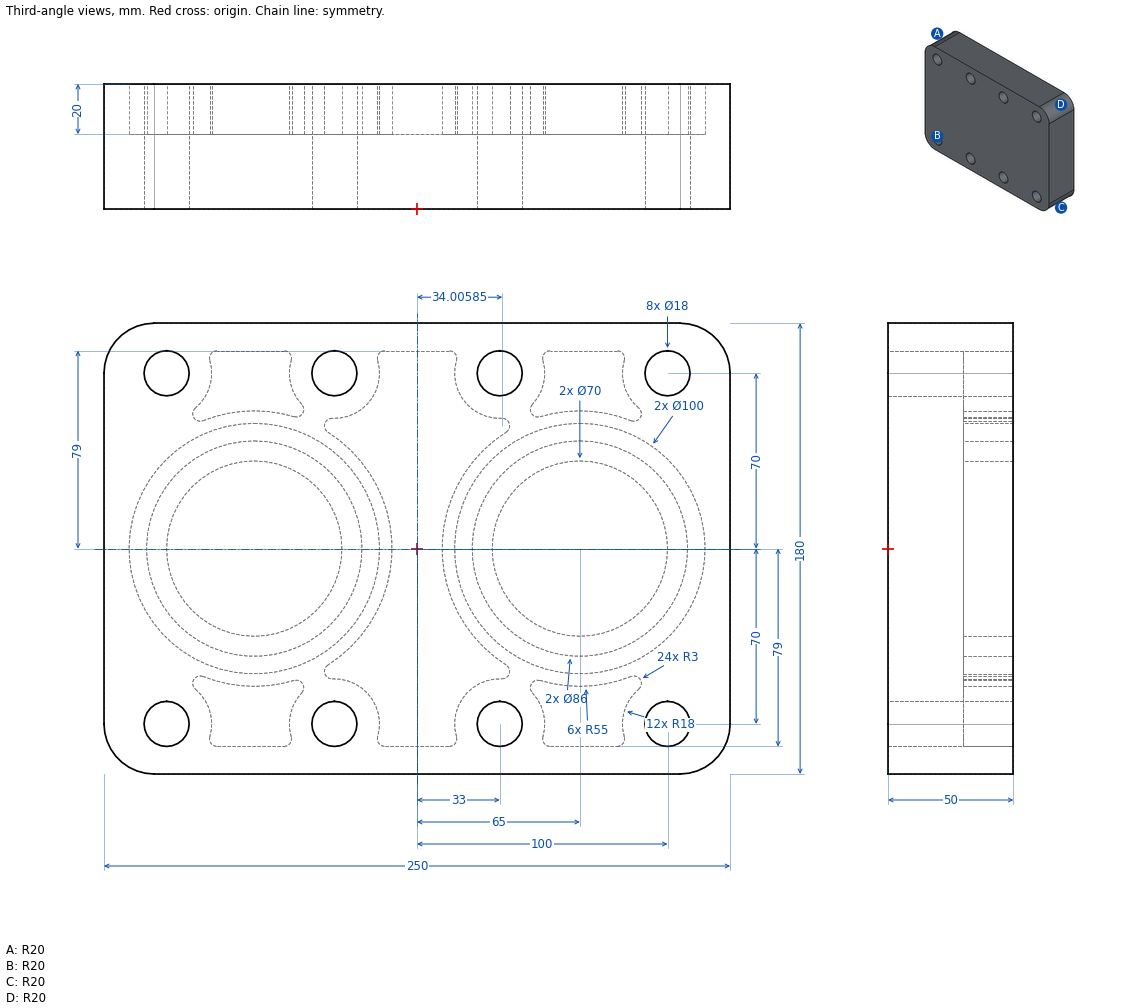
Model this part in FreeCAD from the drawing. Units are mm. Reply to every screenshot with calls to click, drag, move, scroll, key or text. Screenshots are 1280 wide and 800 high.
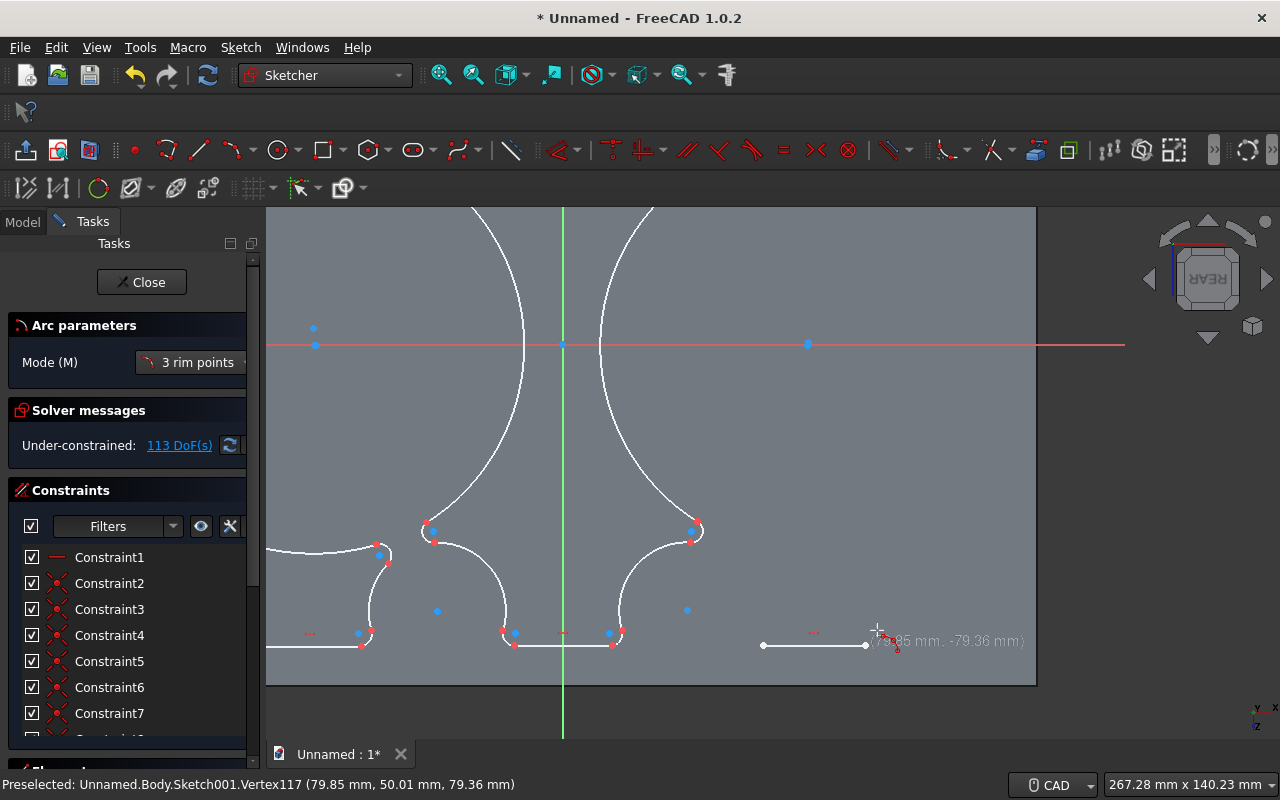
click(877, 630)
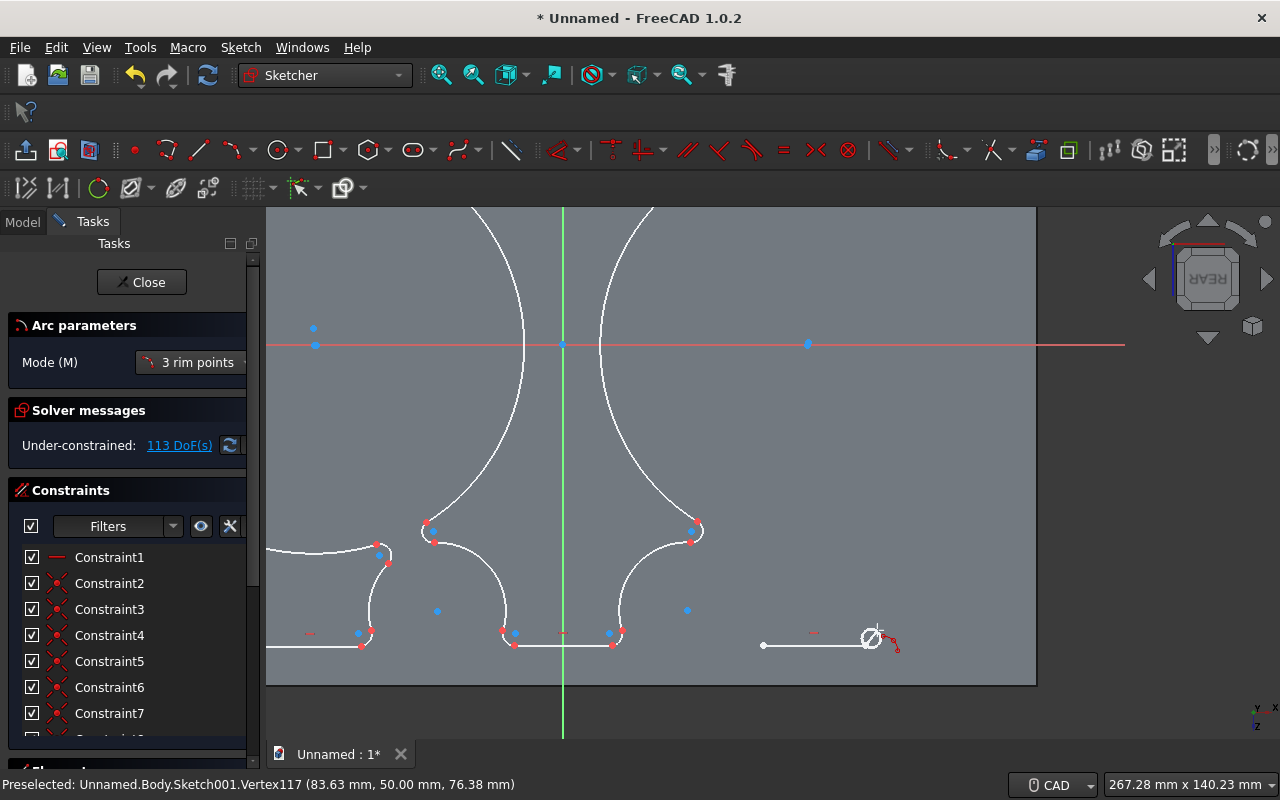
scroll(875, 640, up, 7)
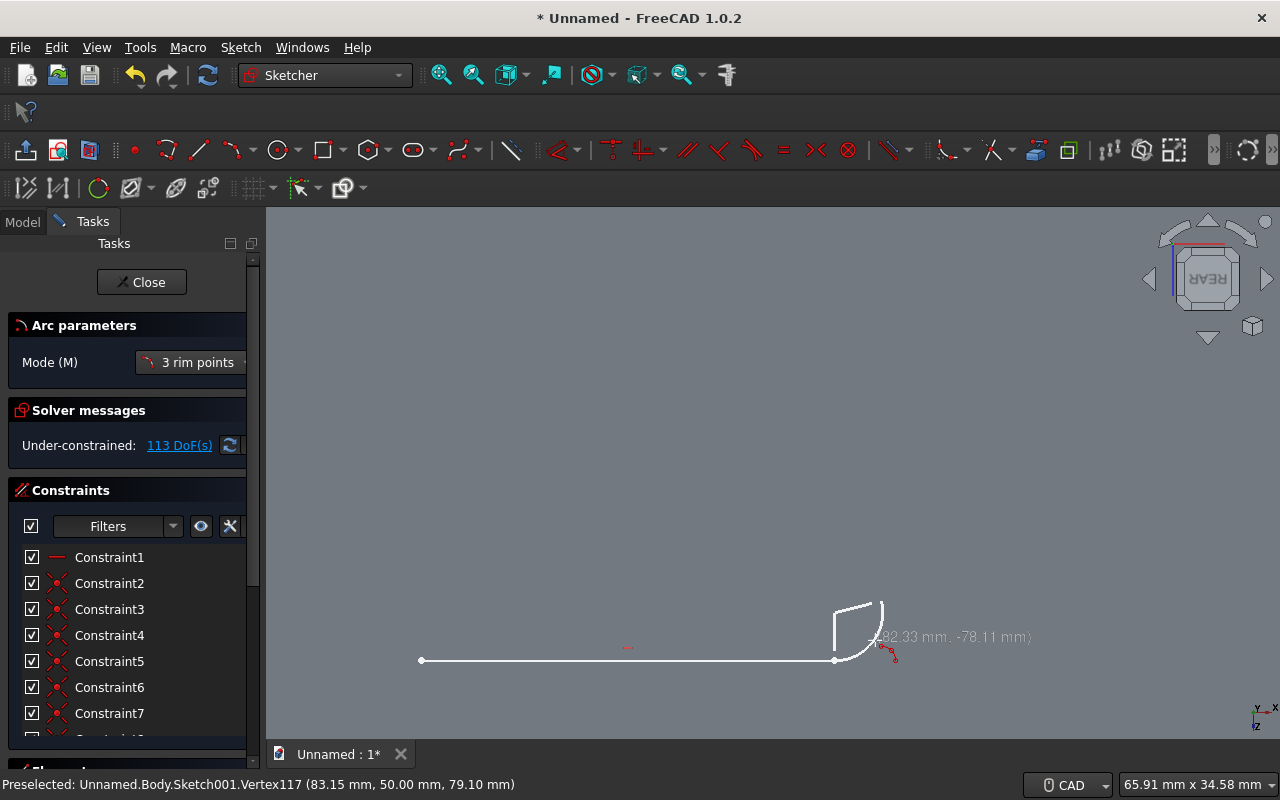
click(872, 637)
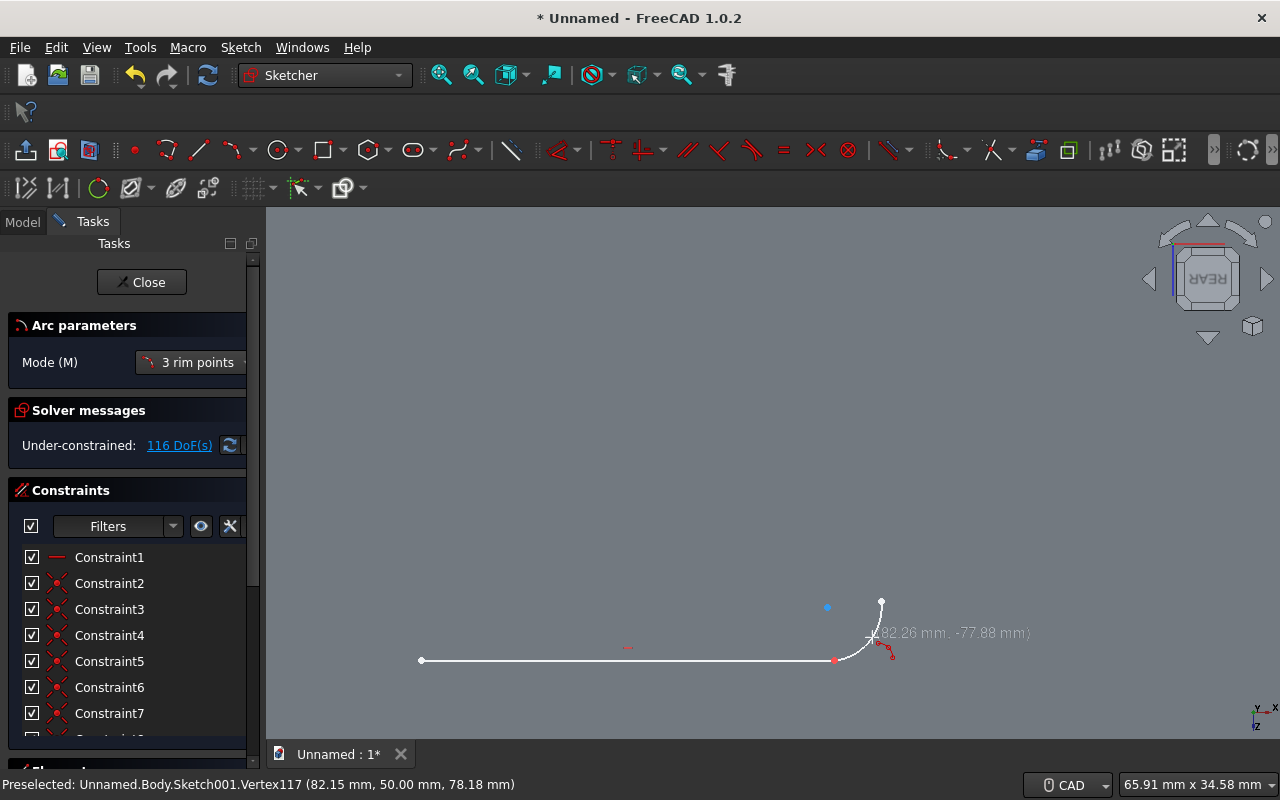
scroll(876, 635, down, 10)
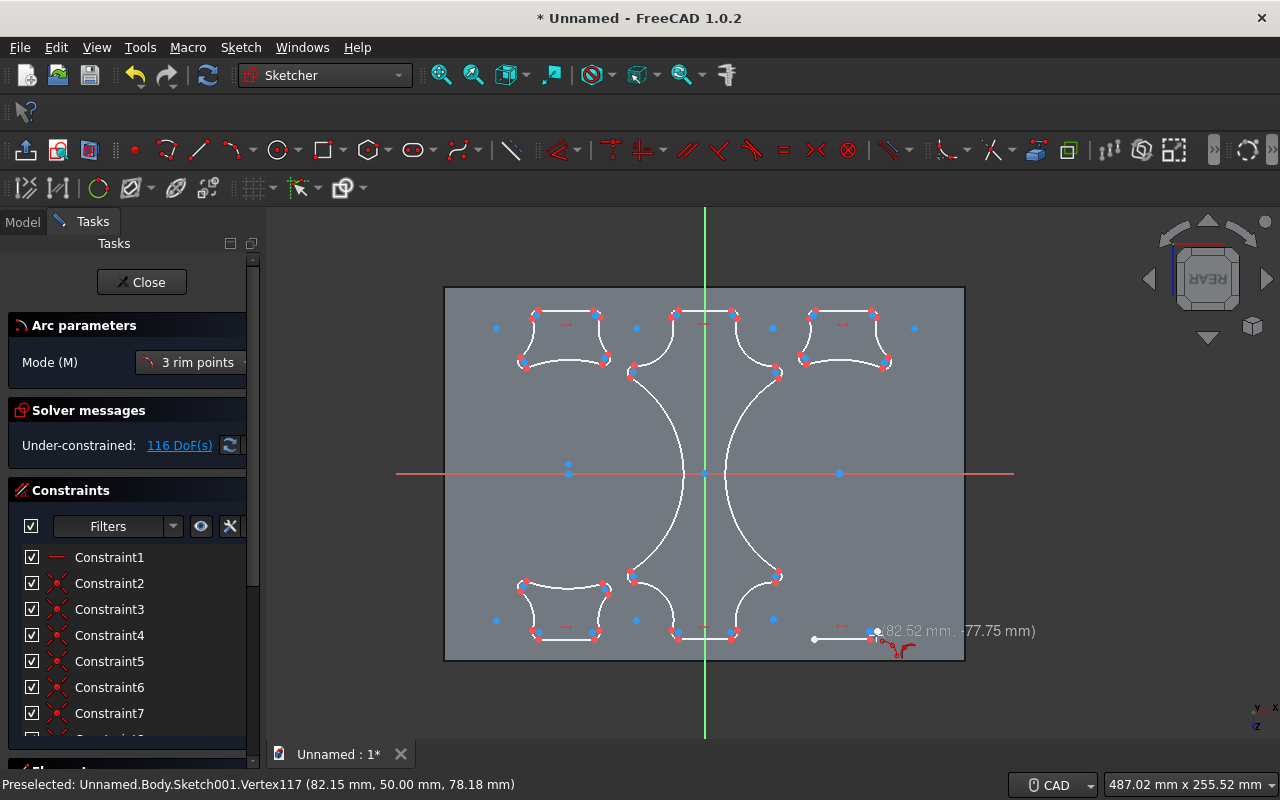
scroll(877, 630, up, 5)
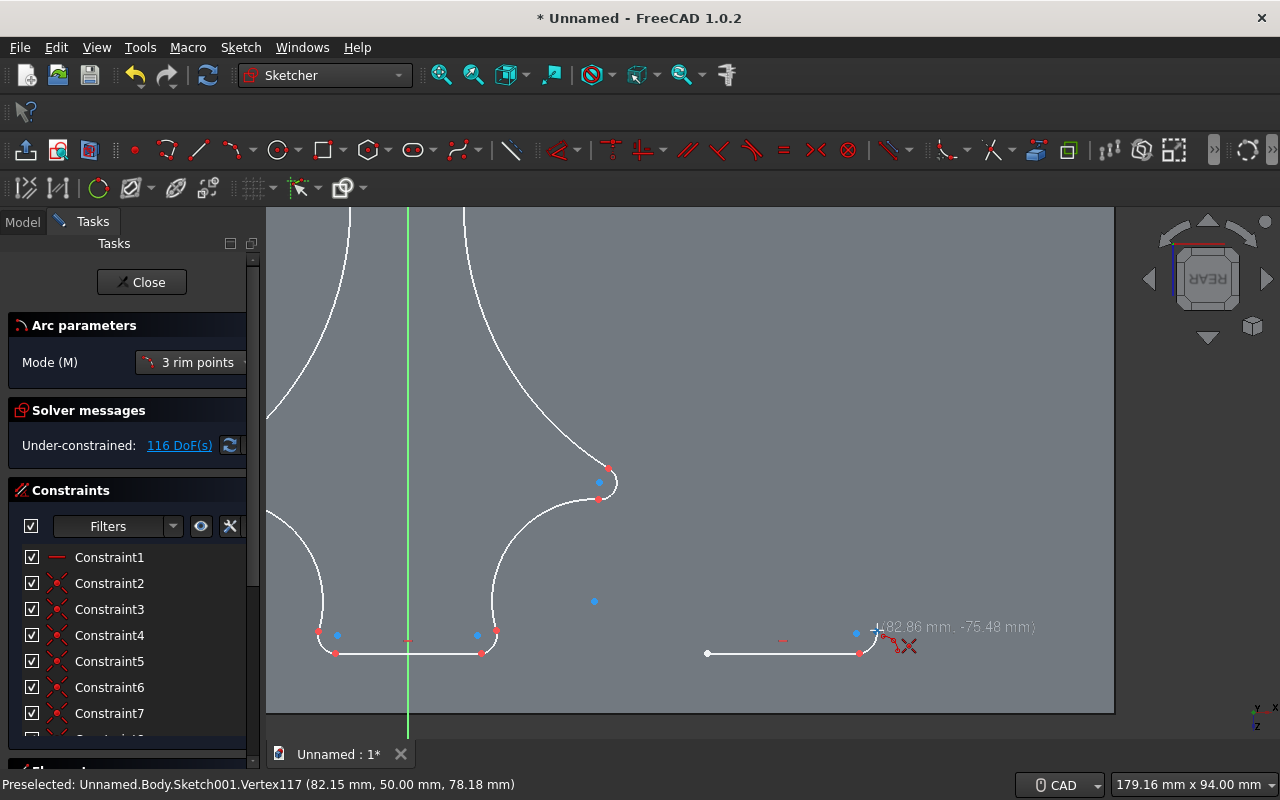
click(877, 632)
click(909, 522)
click(876, 571)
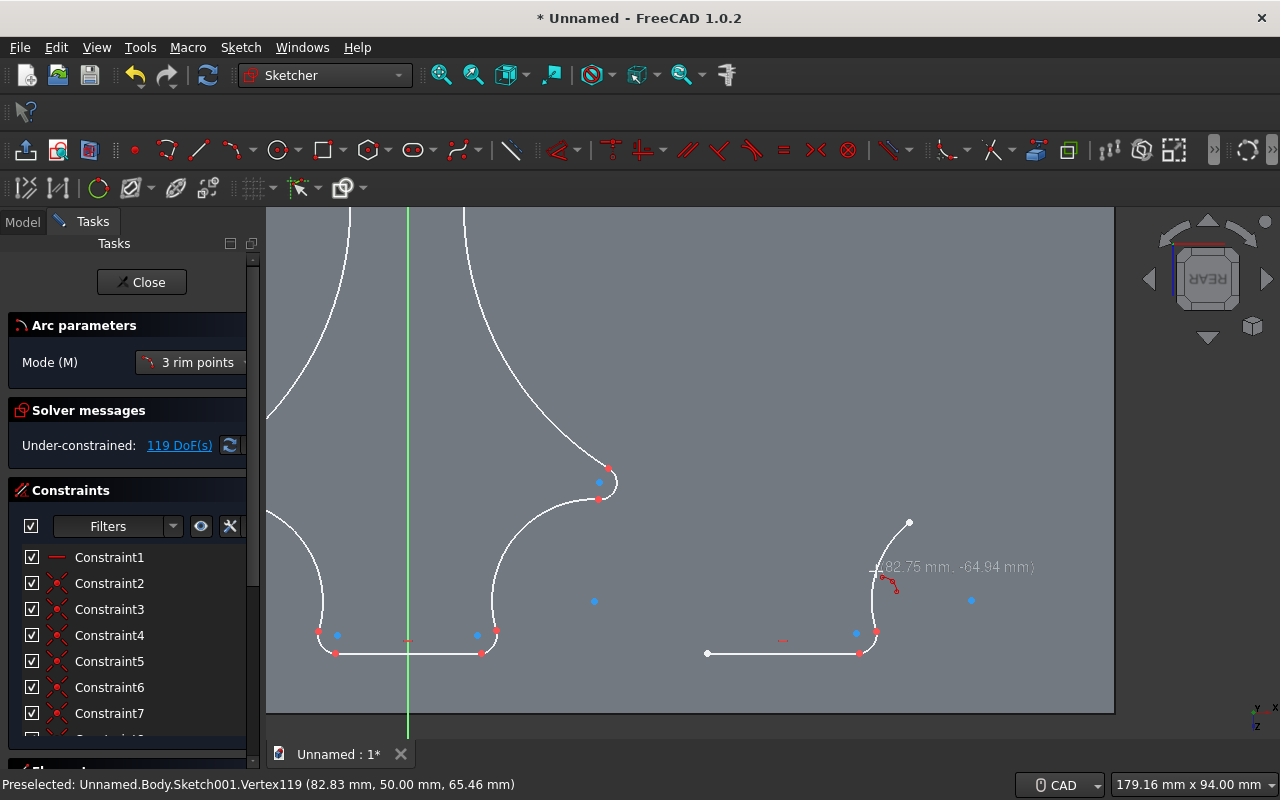
click(909, 523)
click(891, 493)
click(912, 500)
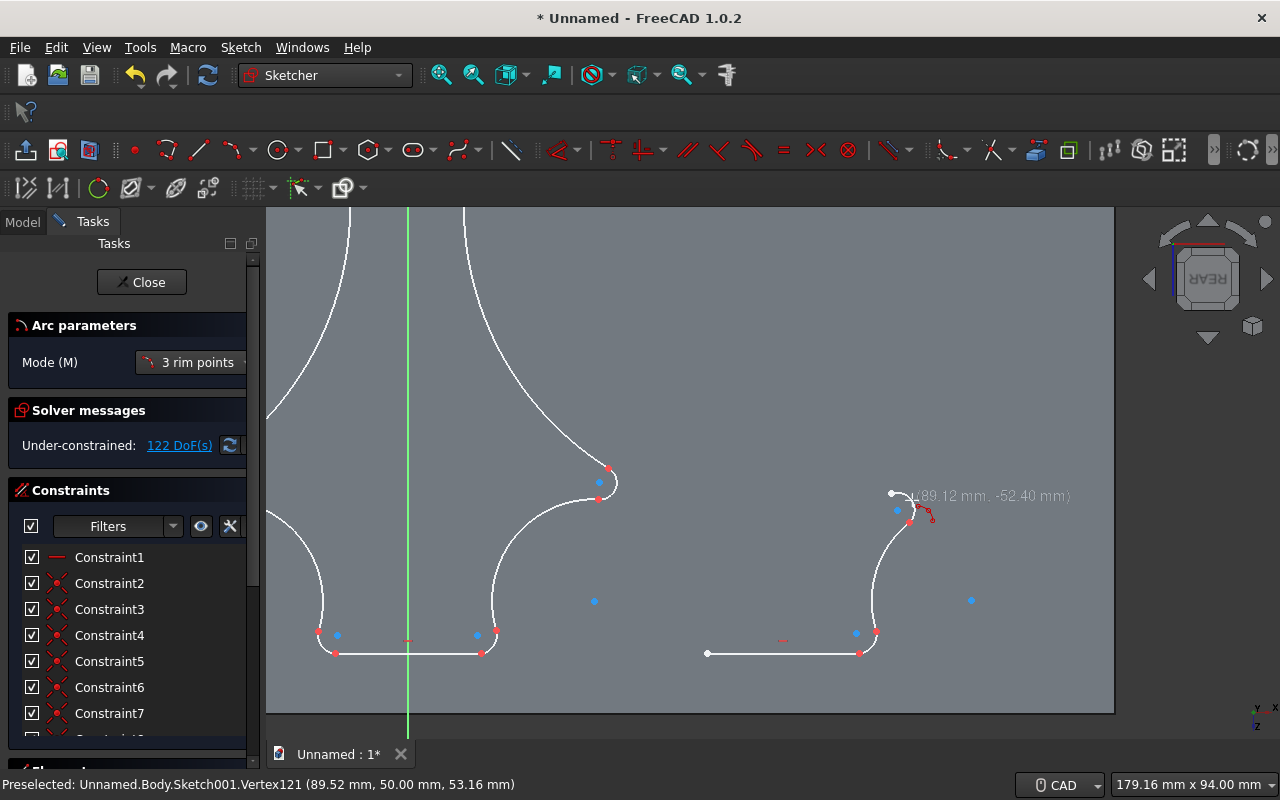
click(891, 494)
click(685, 502)
click(789, 515)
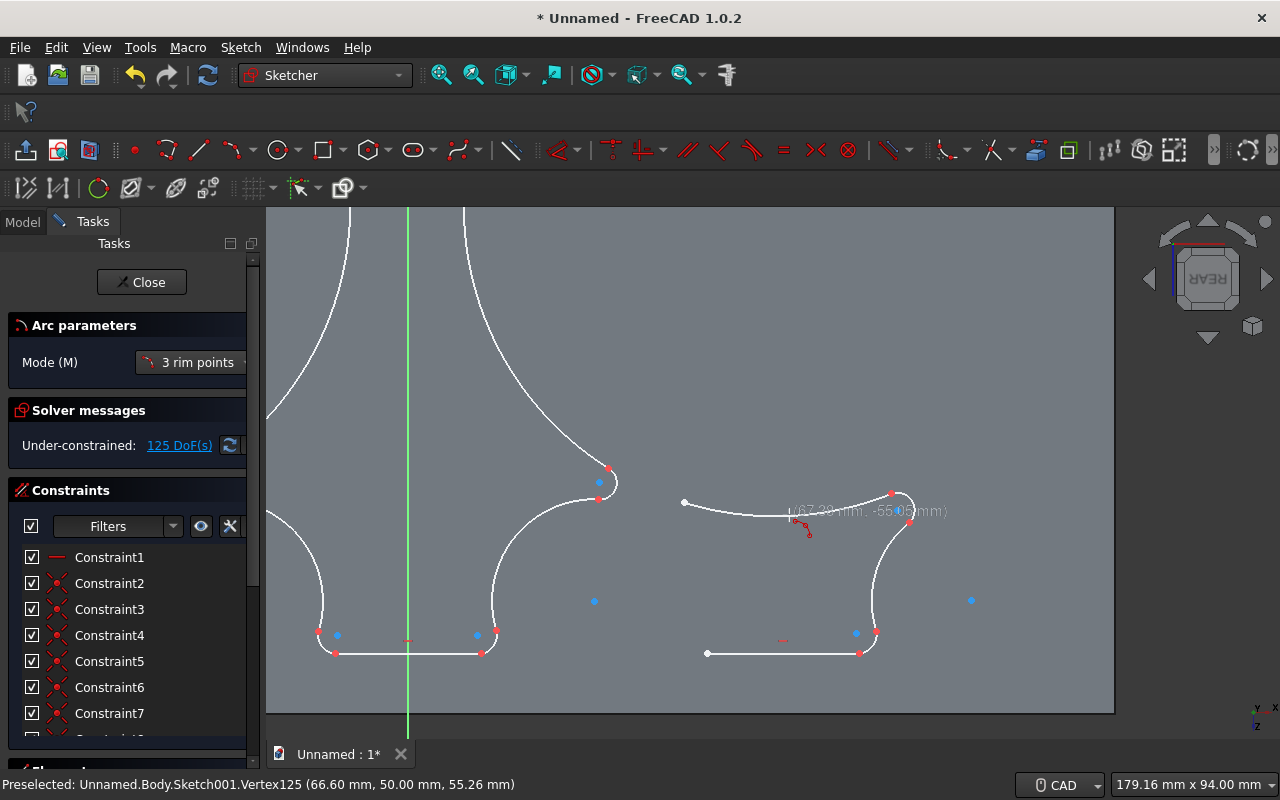
click(685, 503)
click(668, 530)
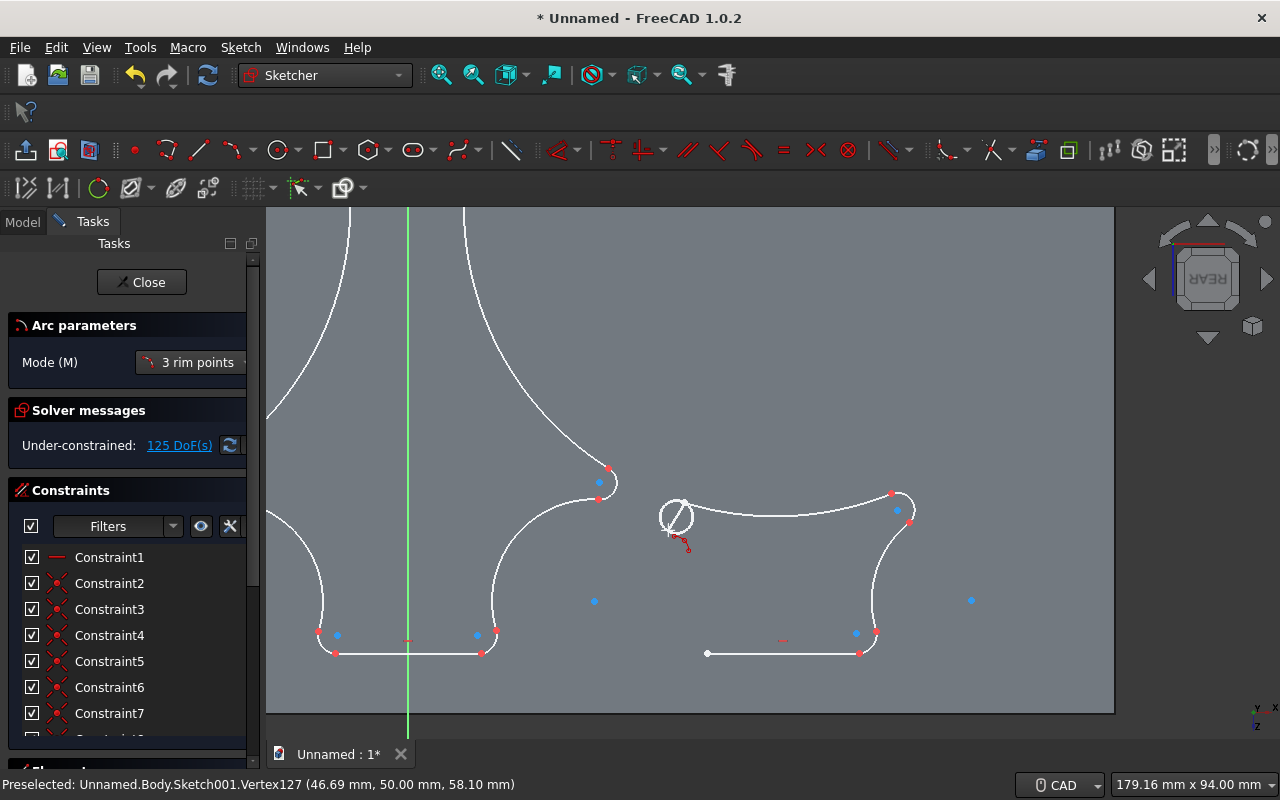
scroll(666, 510, up, 2)